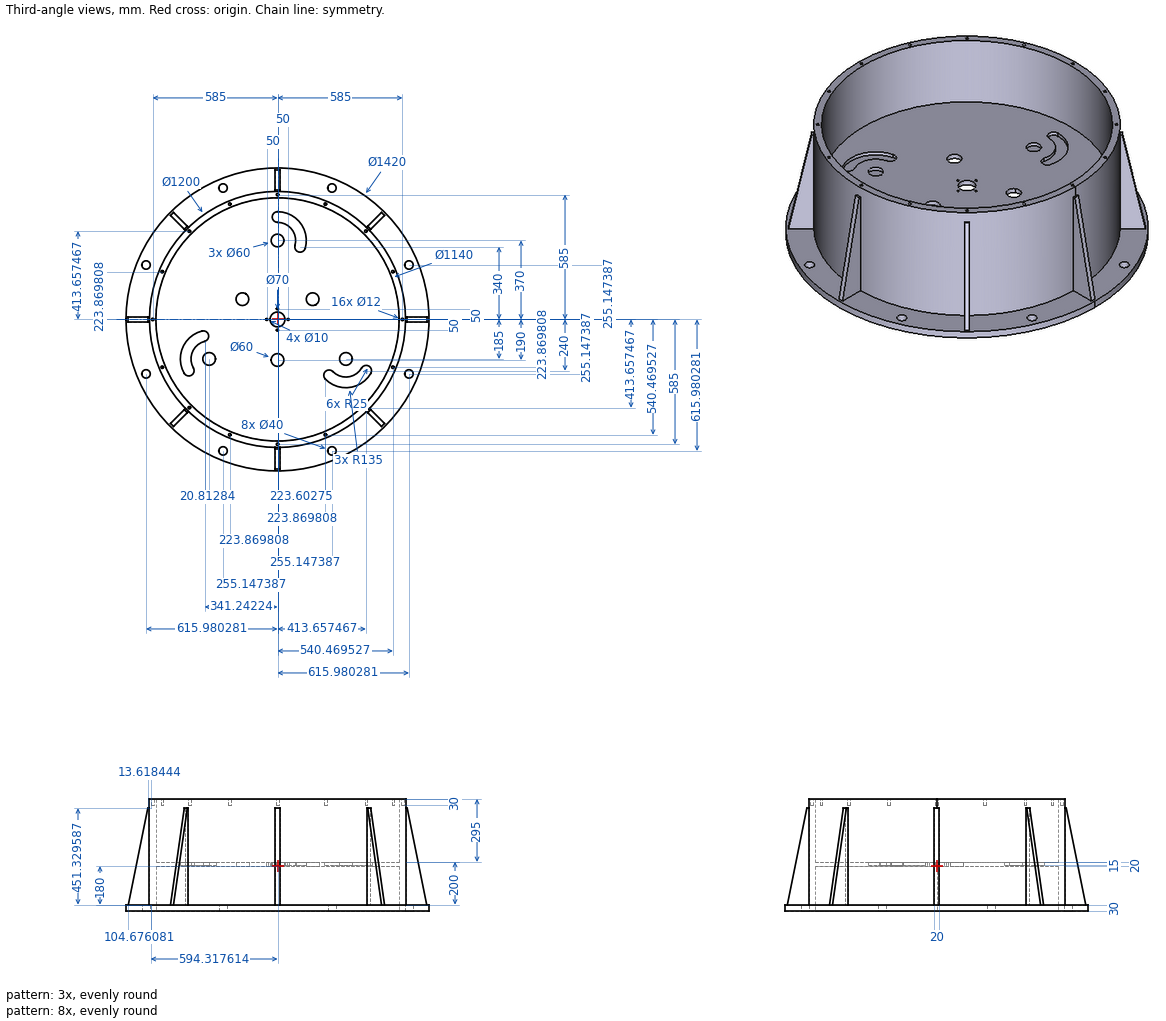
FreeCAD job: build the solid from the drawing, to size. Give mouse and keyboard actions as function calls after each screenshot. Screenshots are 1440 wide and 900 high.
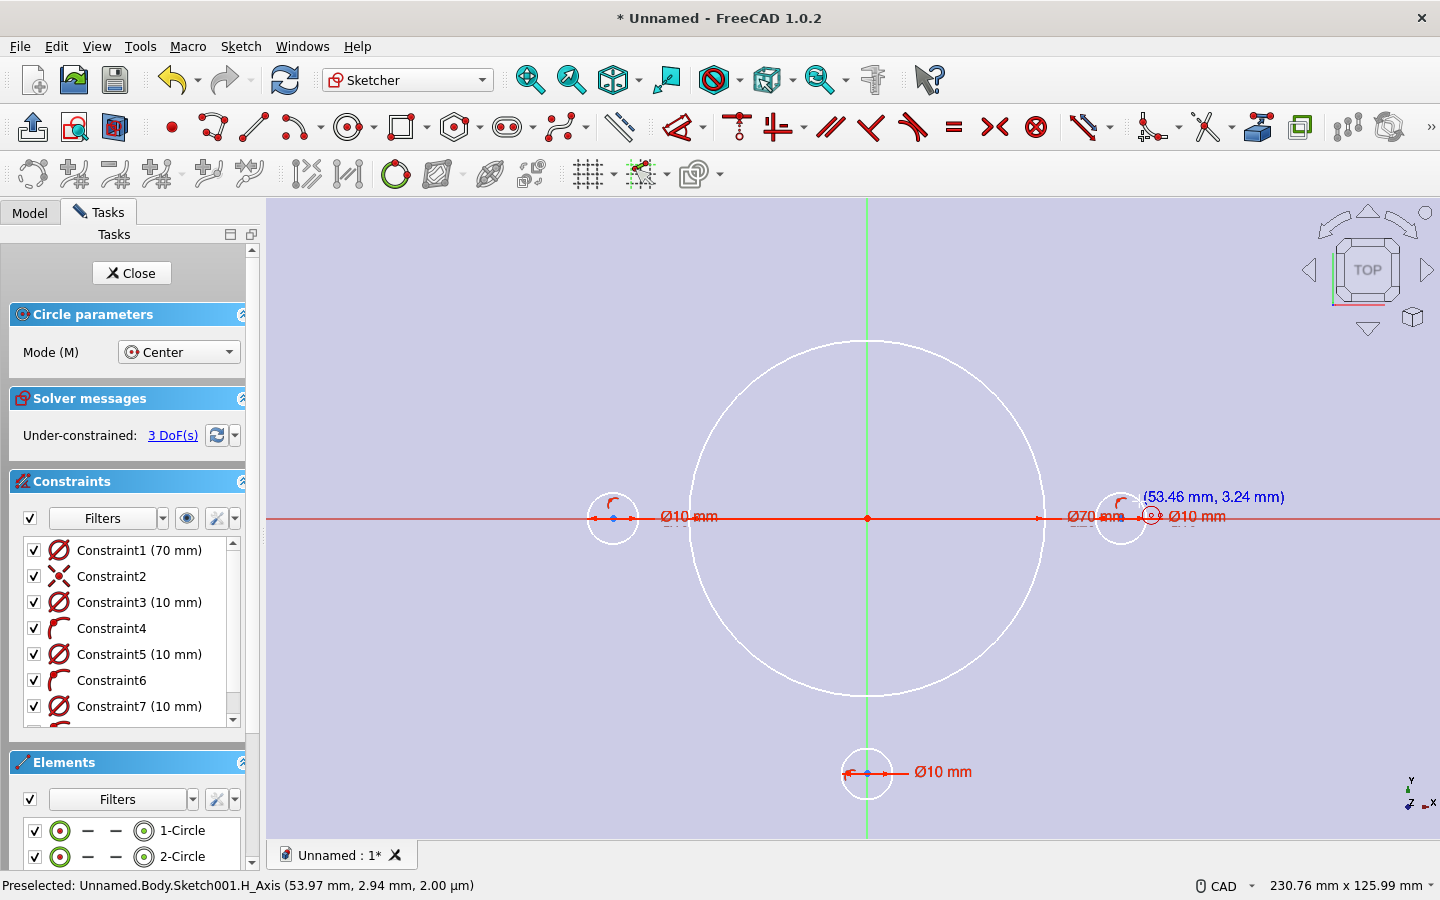
click(867, 264)
move(885, 246)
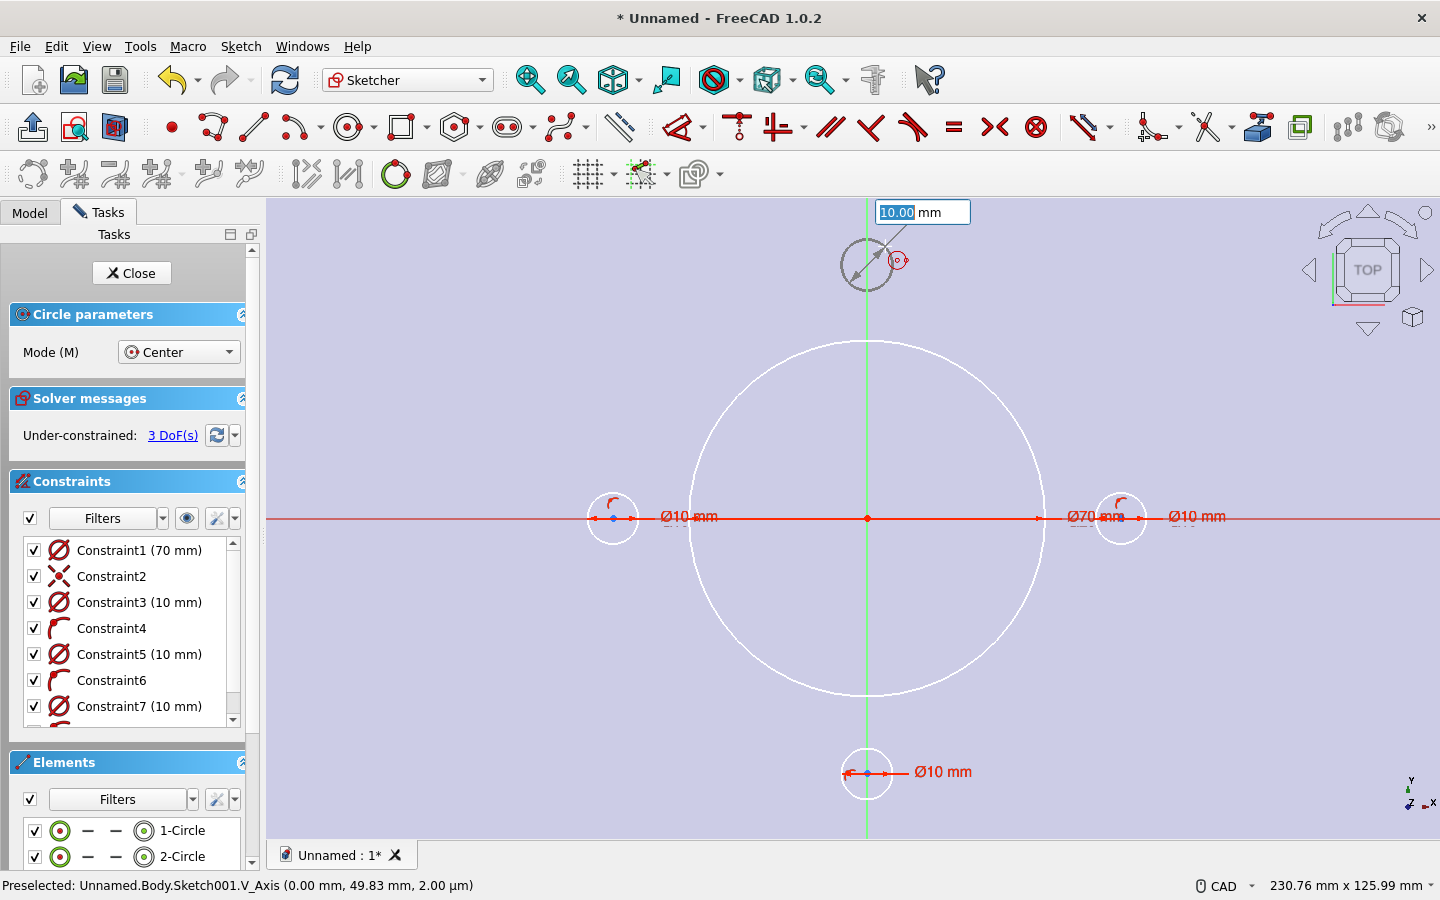
text(10)
key(Return)
key(Escape)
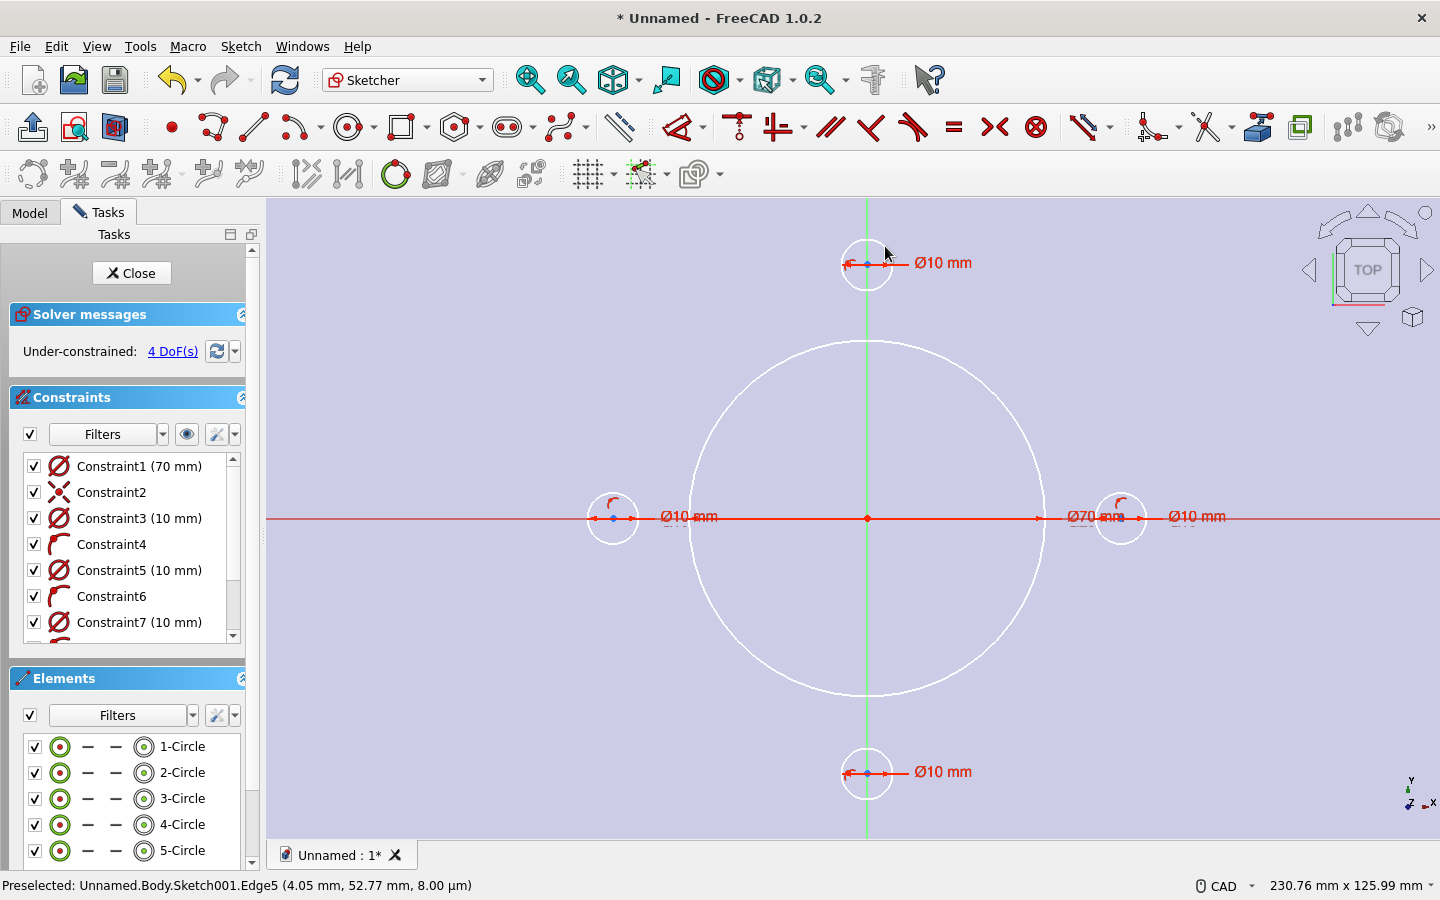
click(613, 518)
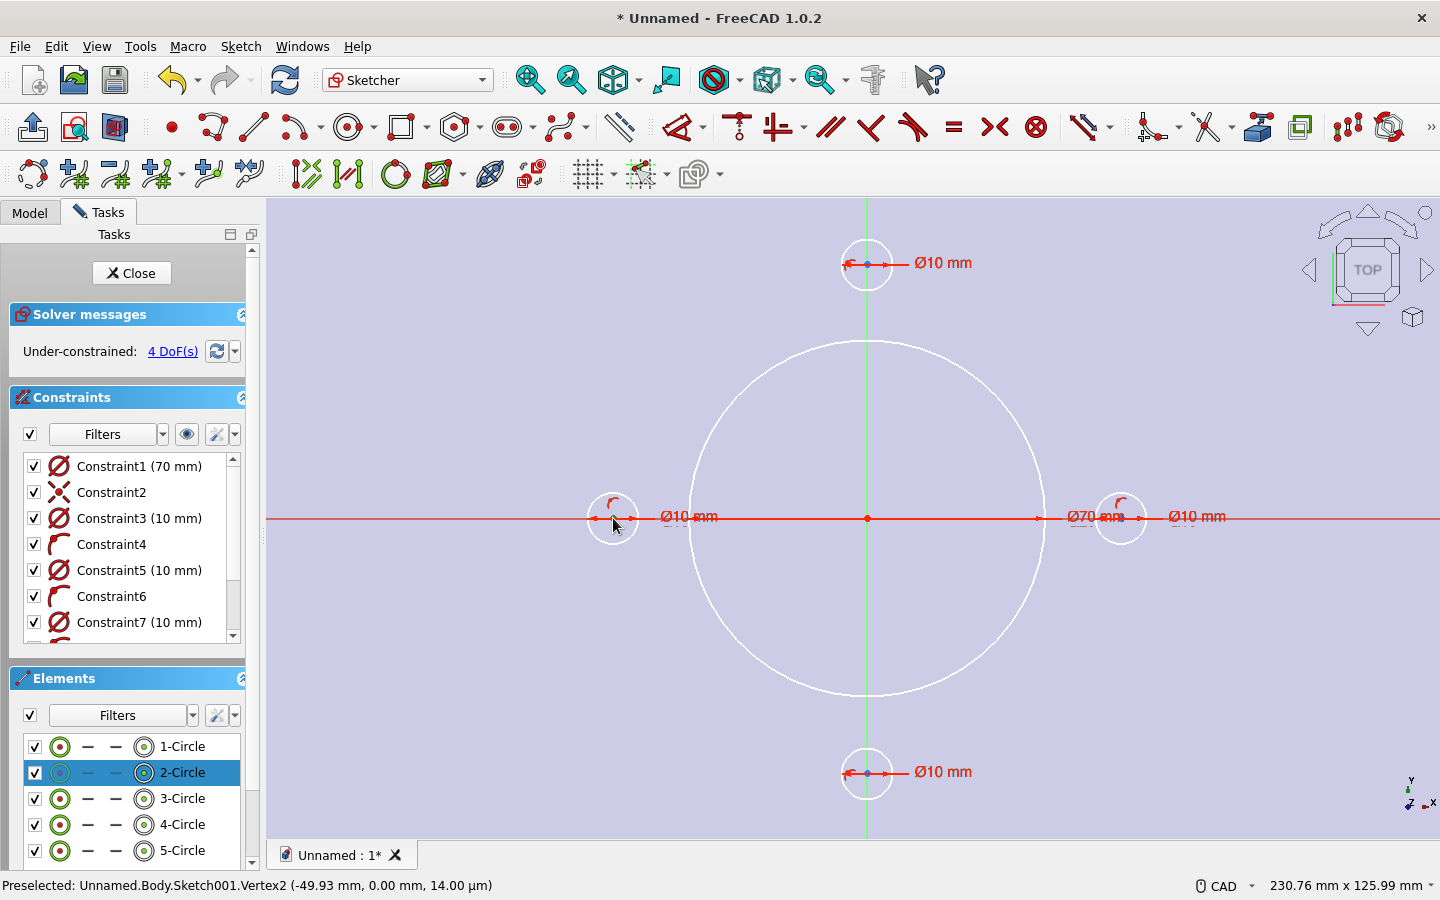
key(l)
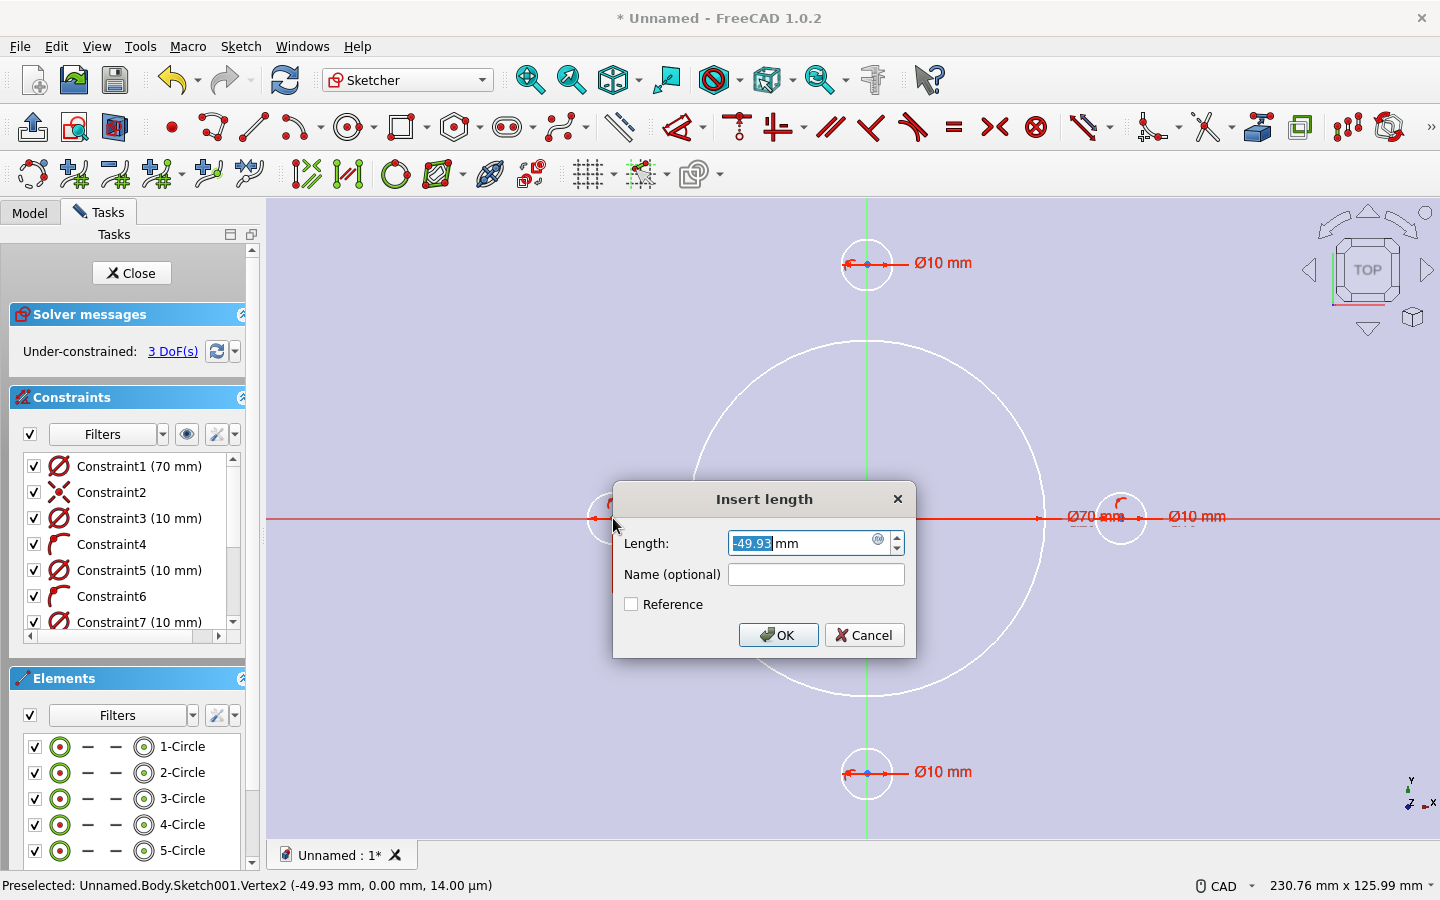
text(-50)
key(Return)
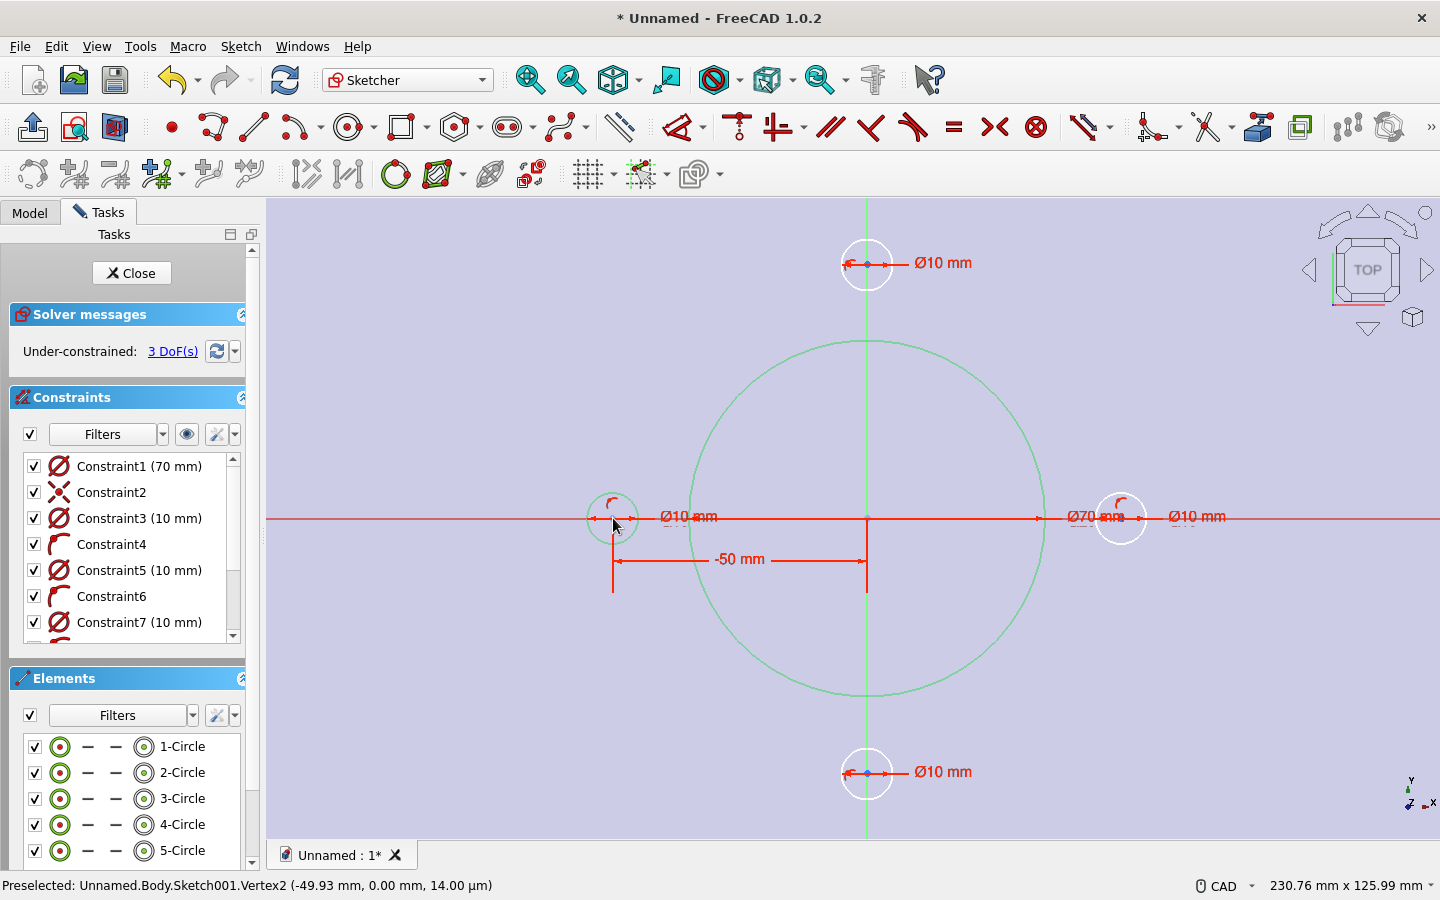
click(867, 774)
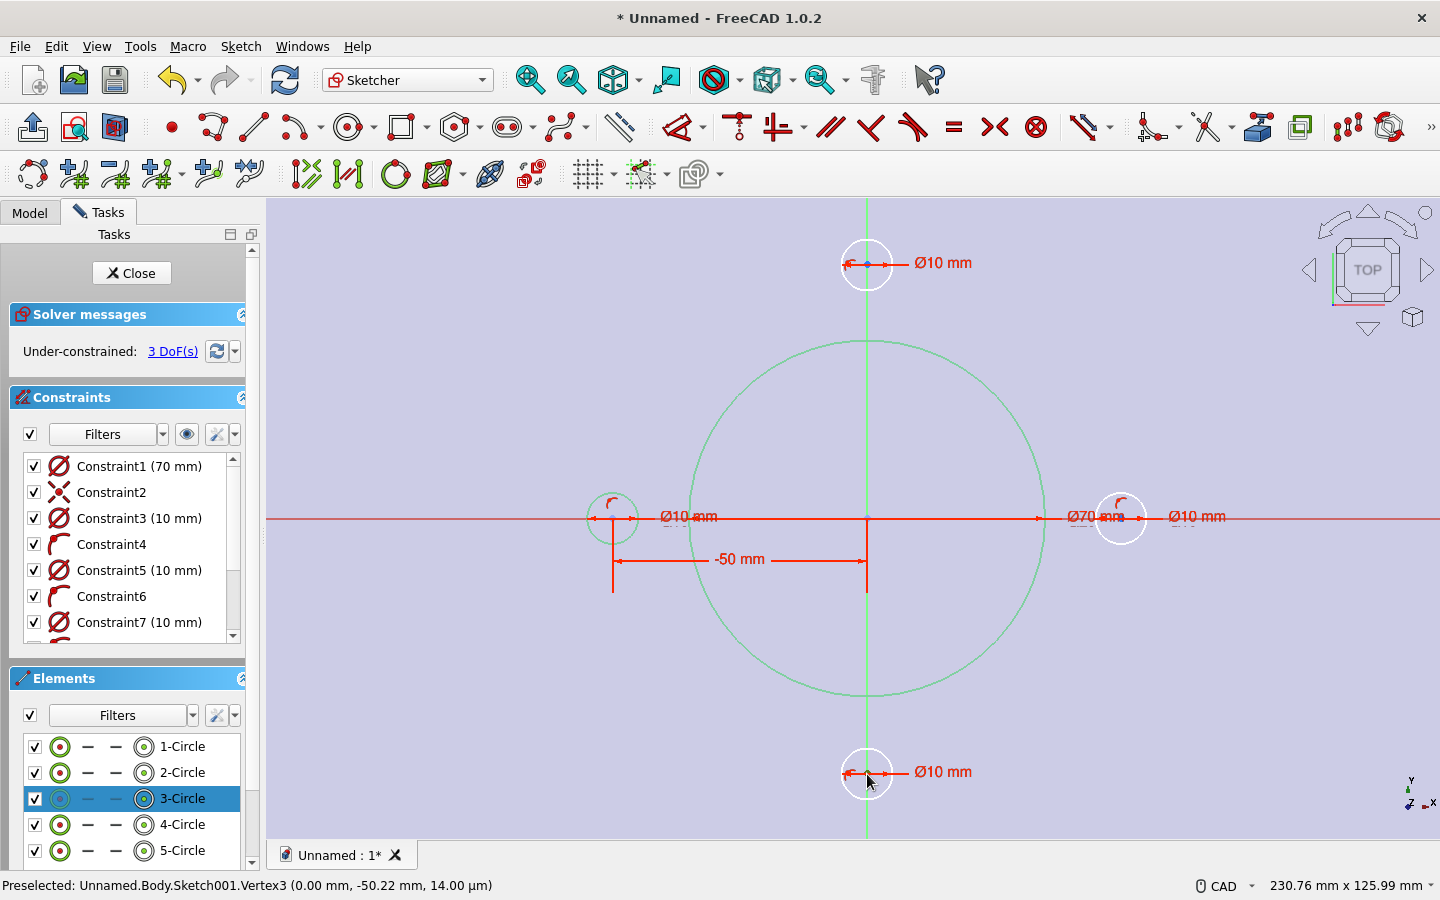
key(i)